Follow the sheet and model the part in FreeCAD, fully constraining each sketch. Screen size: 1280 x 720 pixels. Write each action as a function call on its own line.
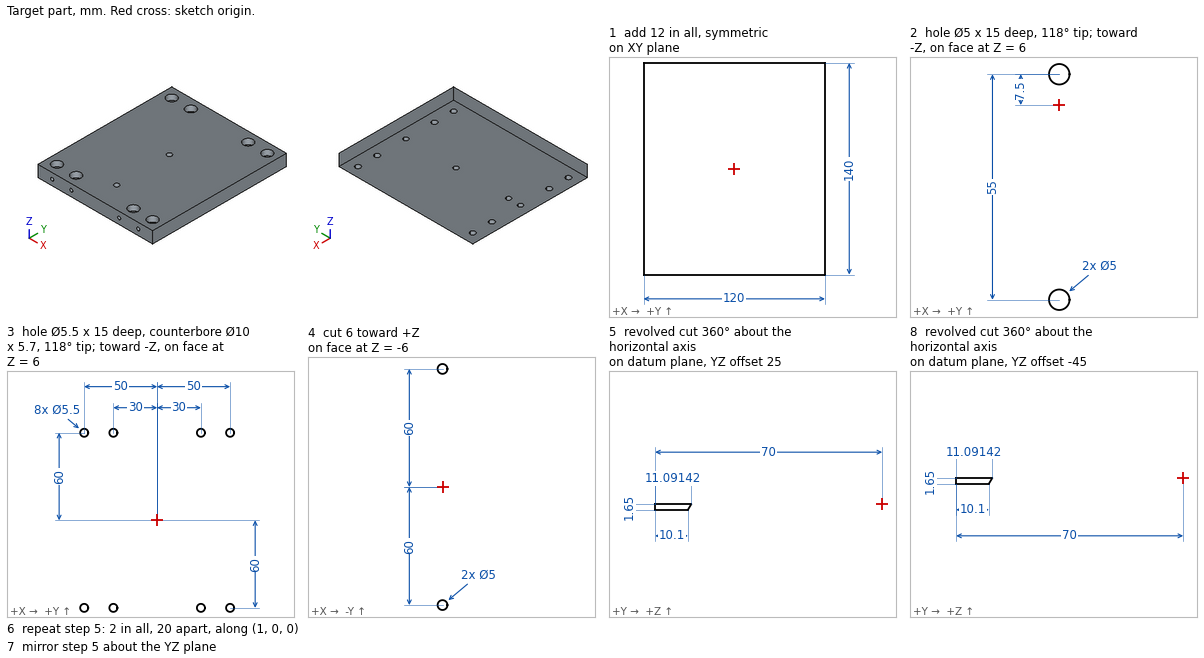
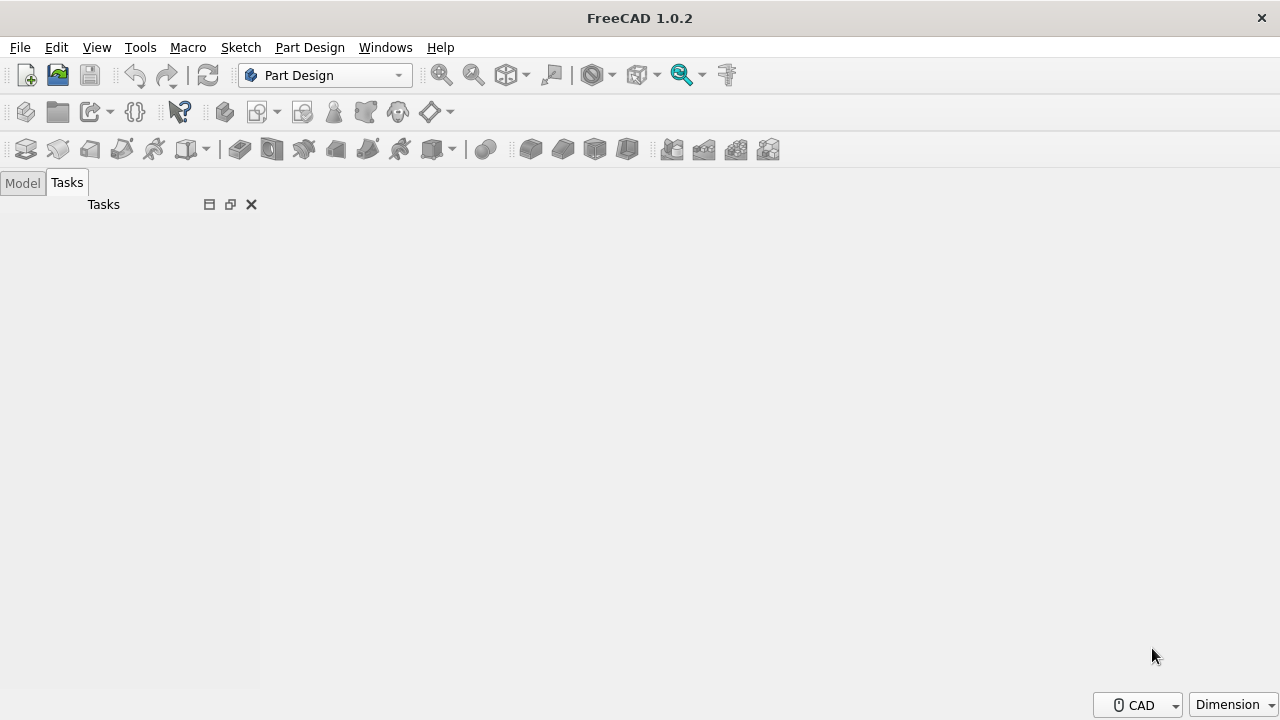
click(26, 76)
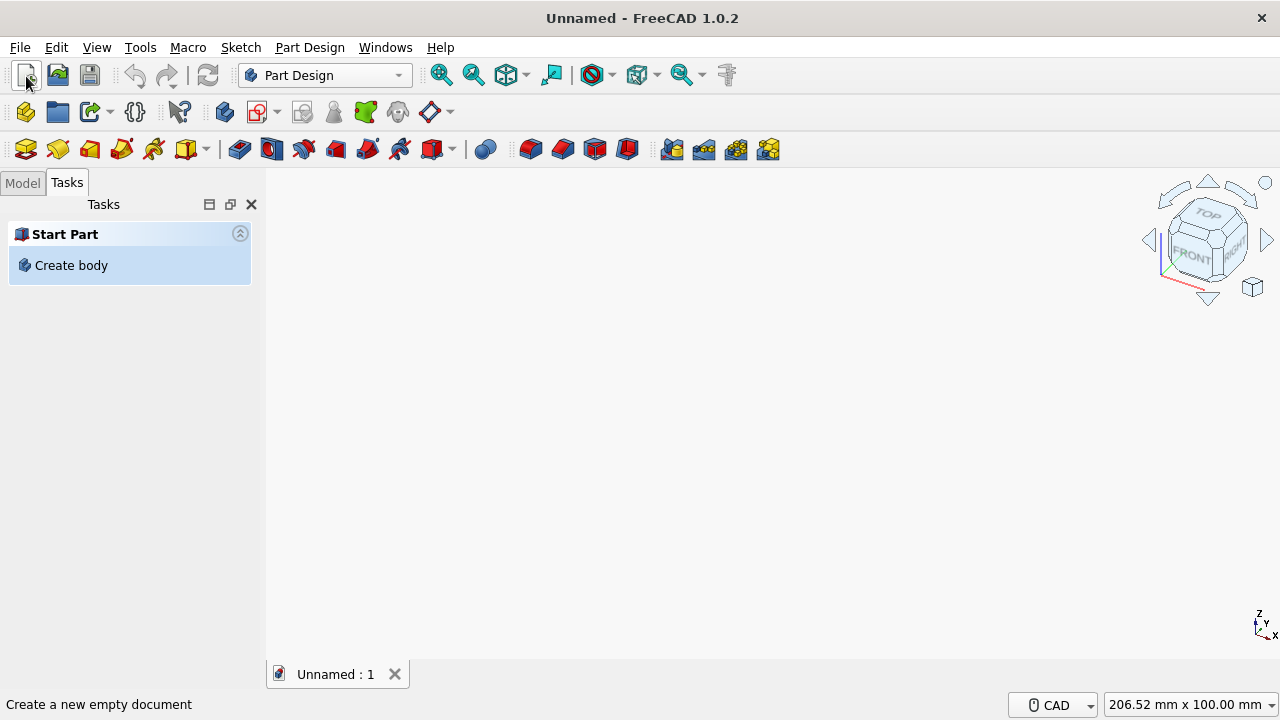
click(258, 112)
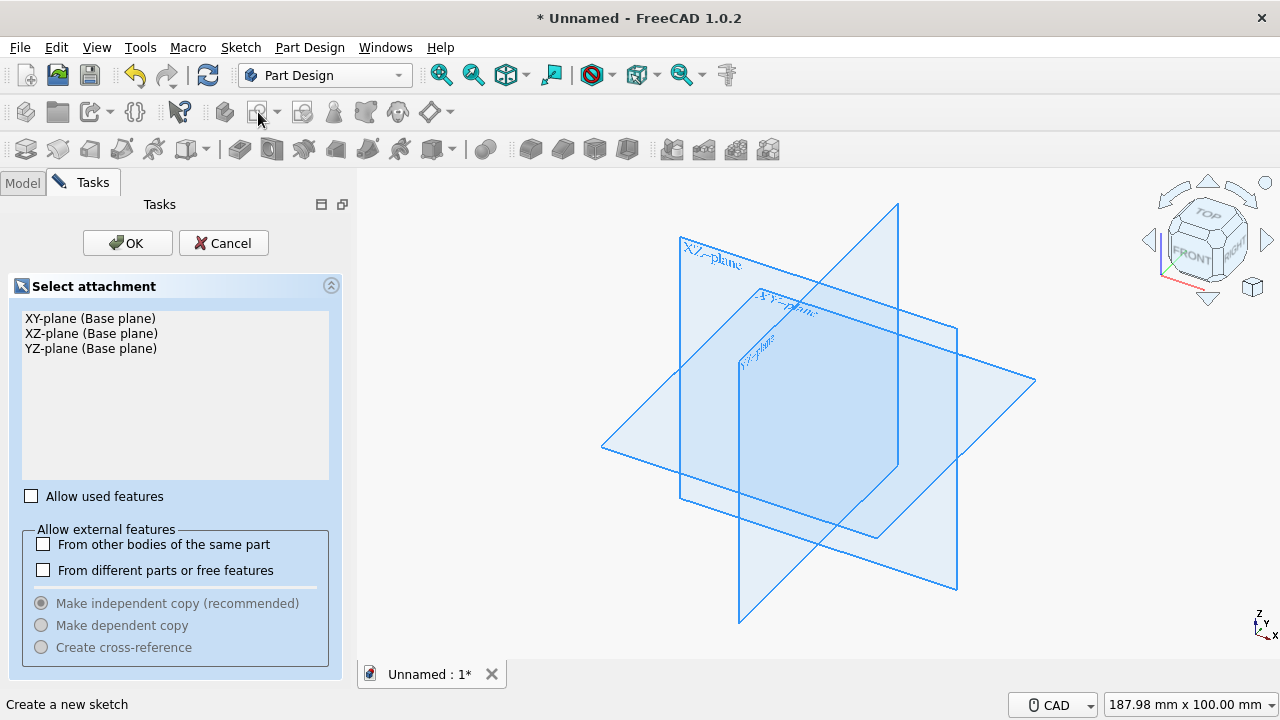
click(82, 318)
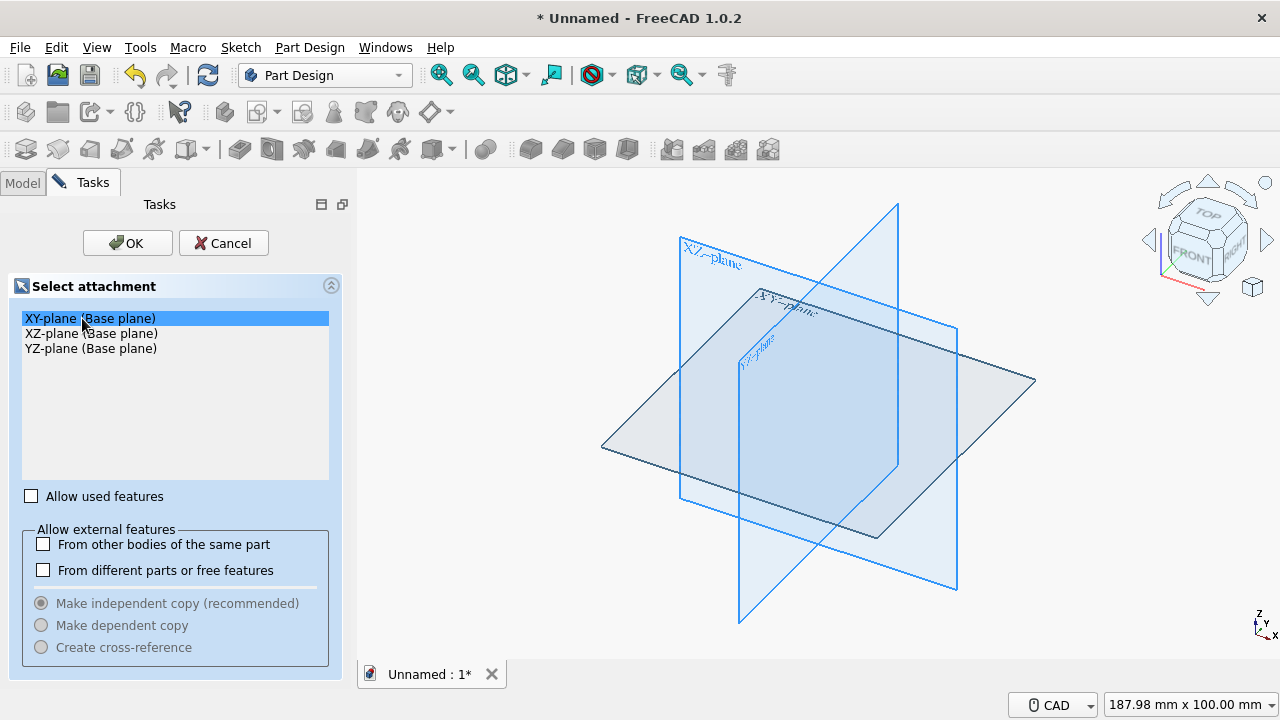
click(128, 243)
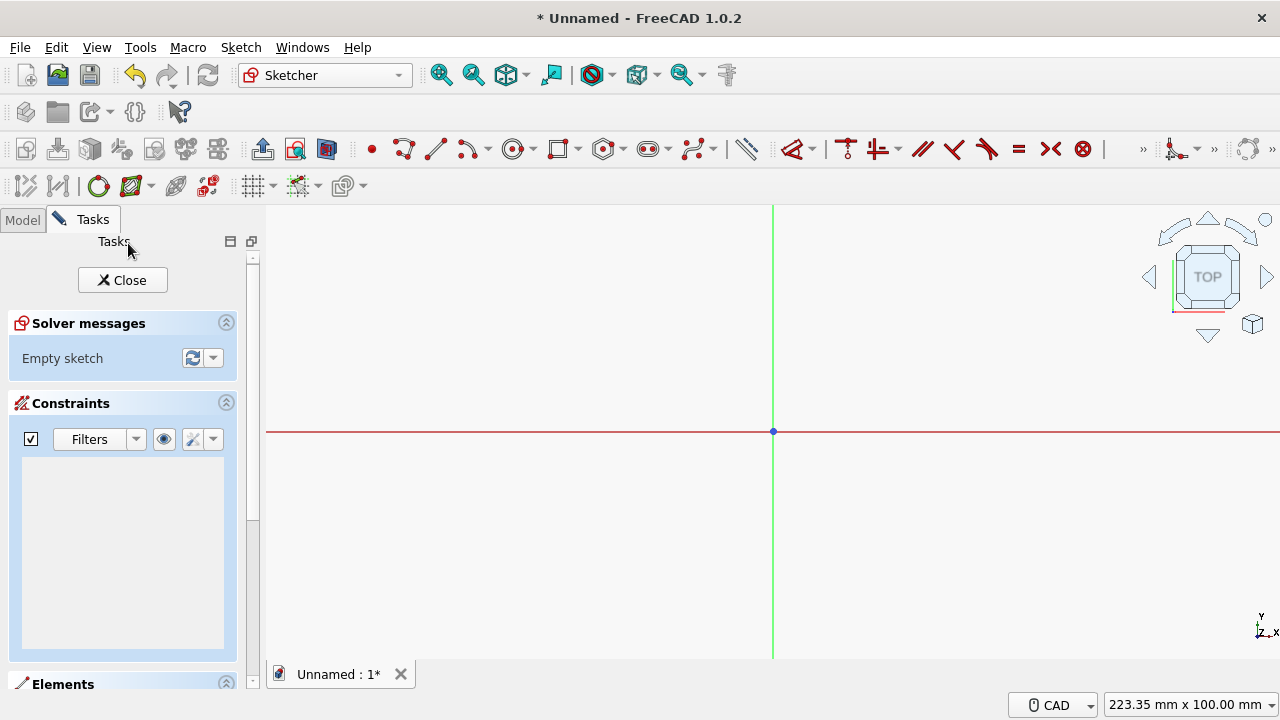
scroll(649, 432, down, 4)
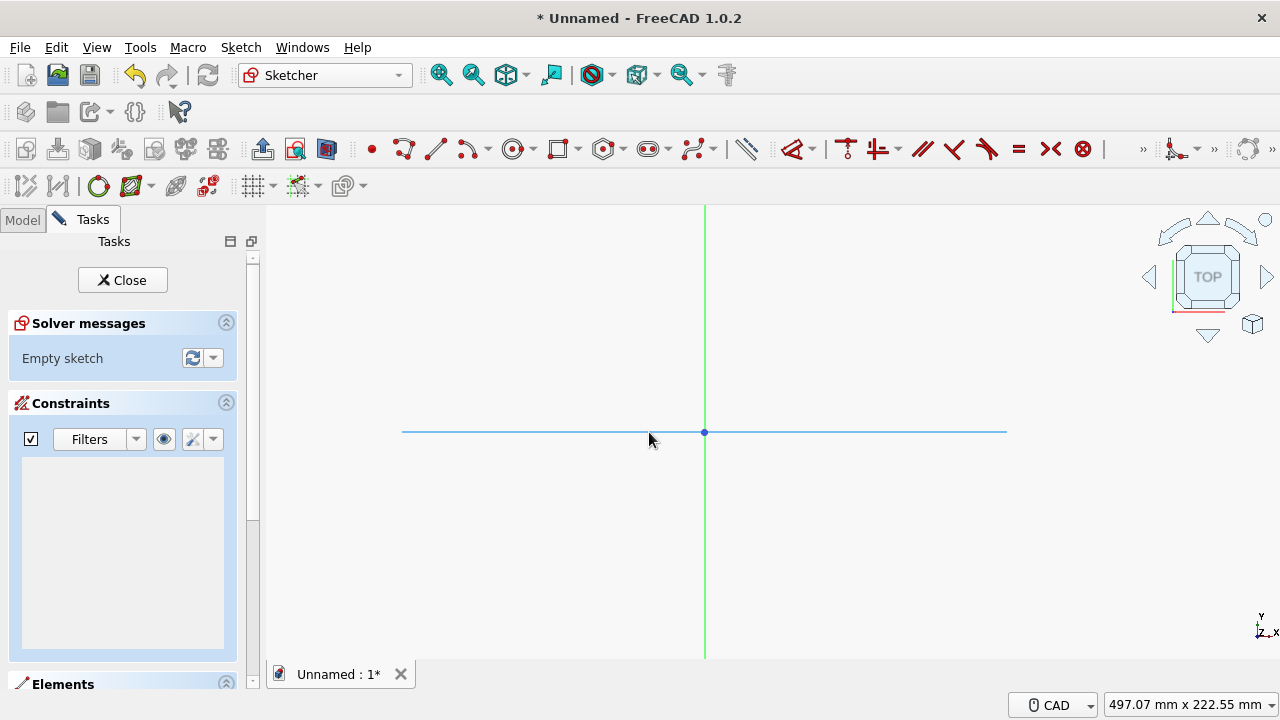
click(580, 150)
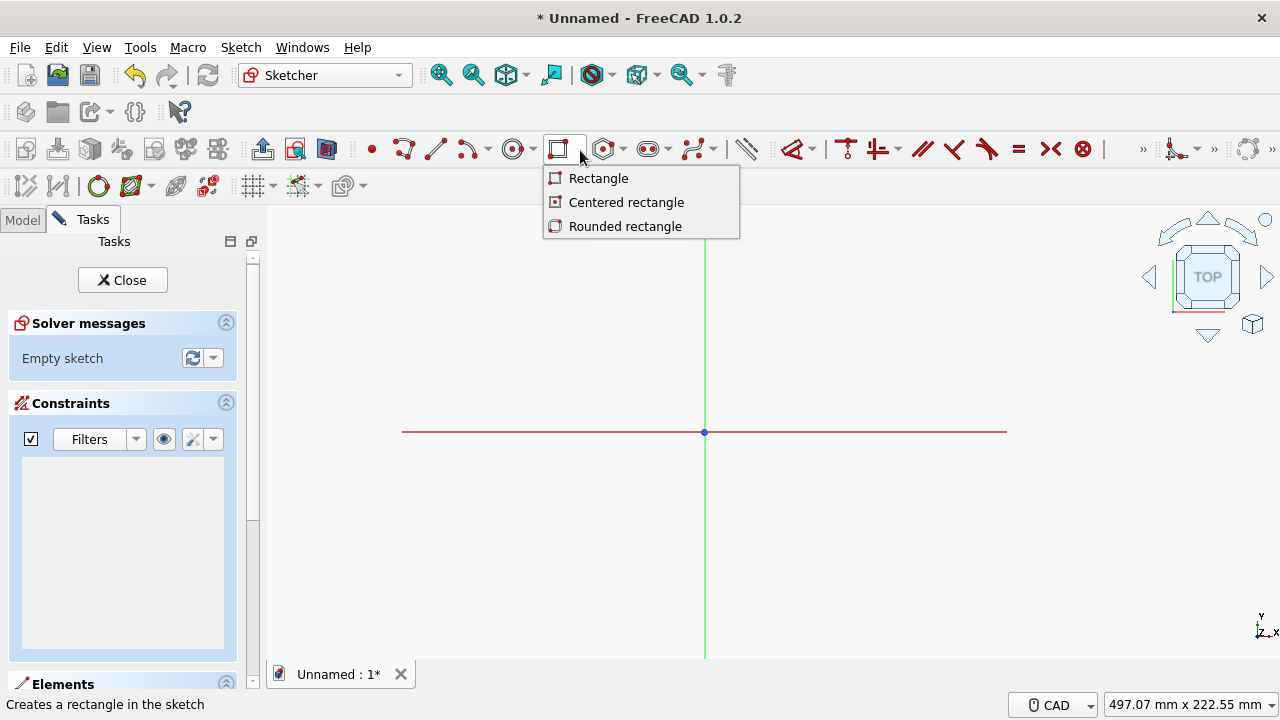
click(642, 202)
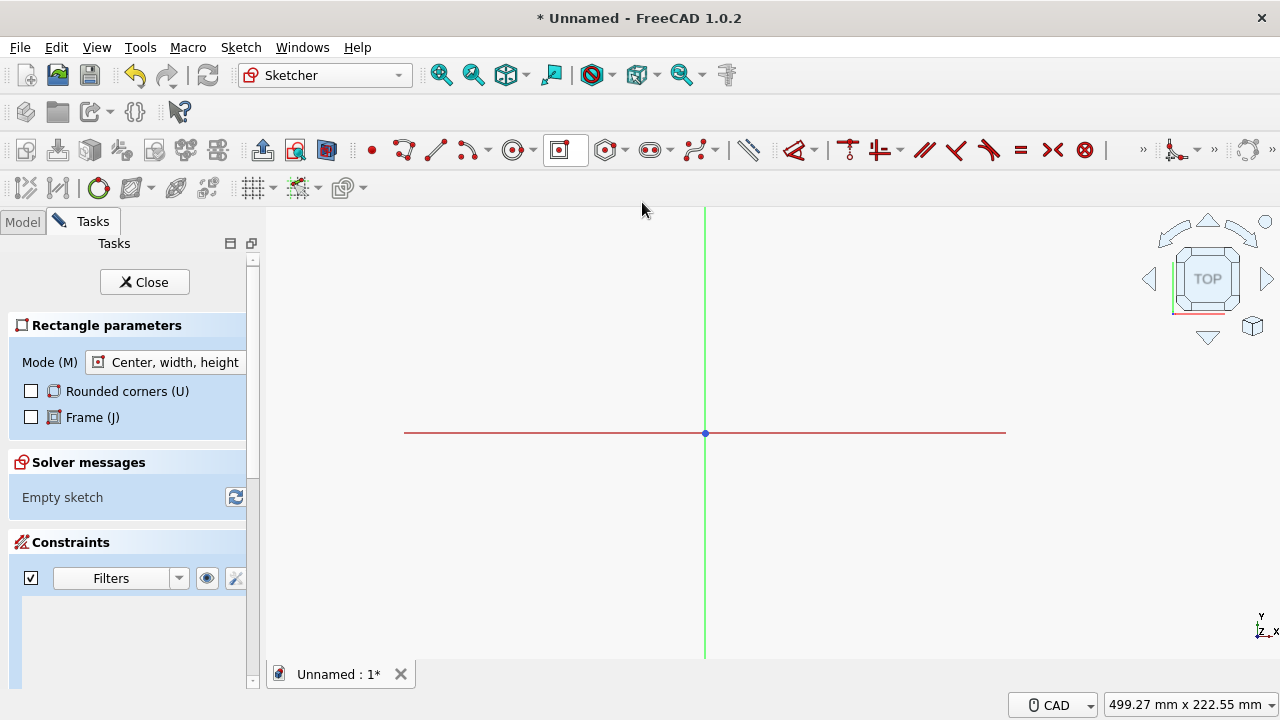
click(705, 433)
move(827, 291)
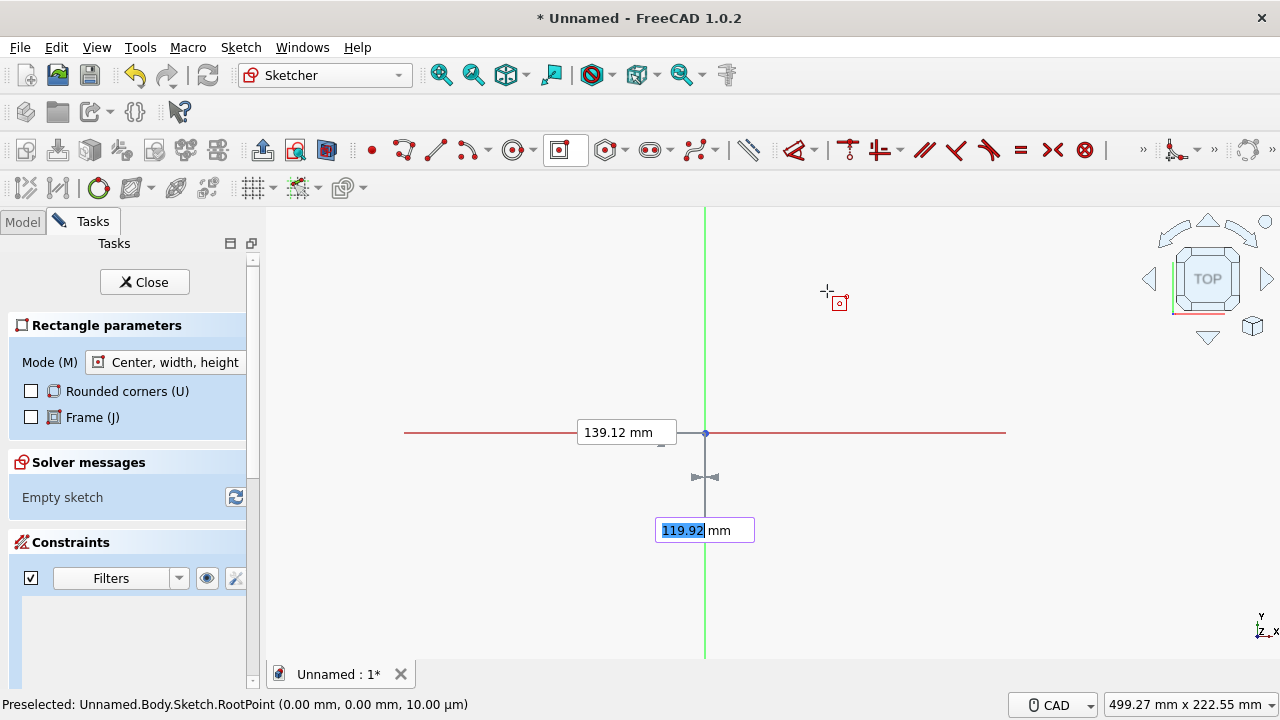
text(120)
key(Tab)
text(140)
key(Return)
key(Escape)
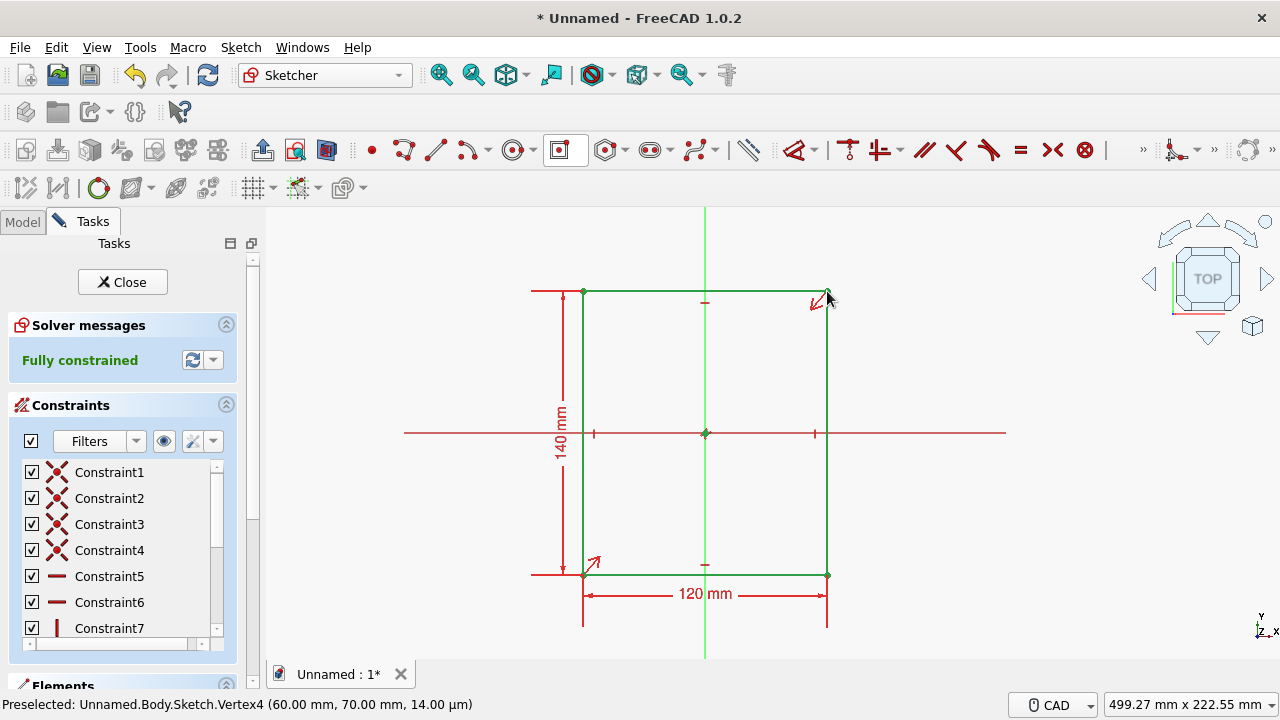
click(123, 282)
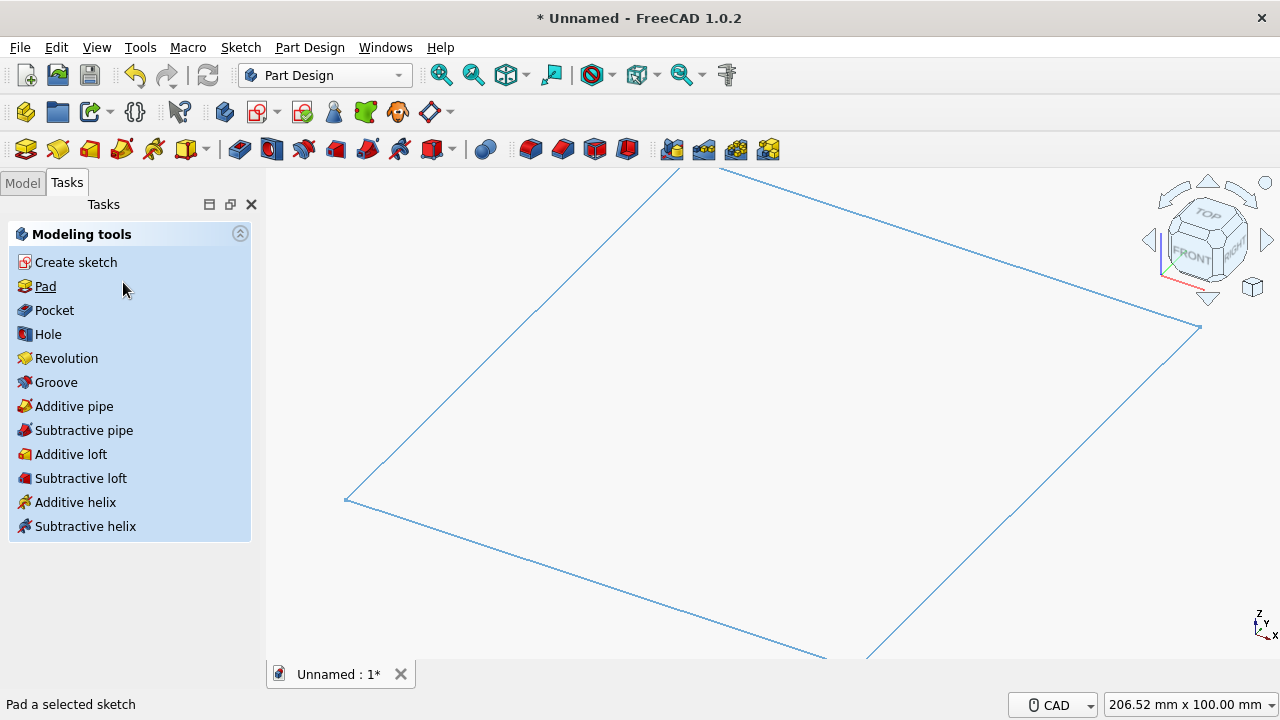
click(26, 150)